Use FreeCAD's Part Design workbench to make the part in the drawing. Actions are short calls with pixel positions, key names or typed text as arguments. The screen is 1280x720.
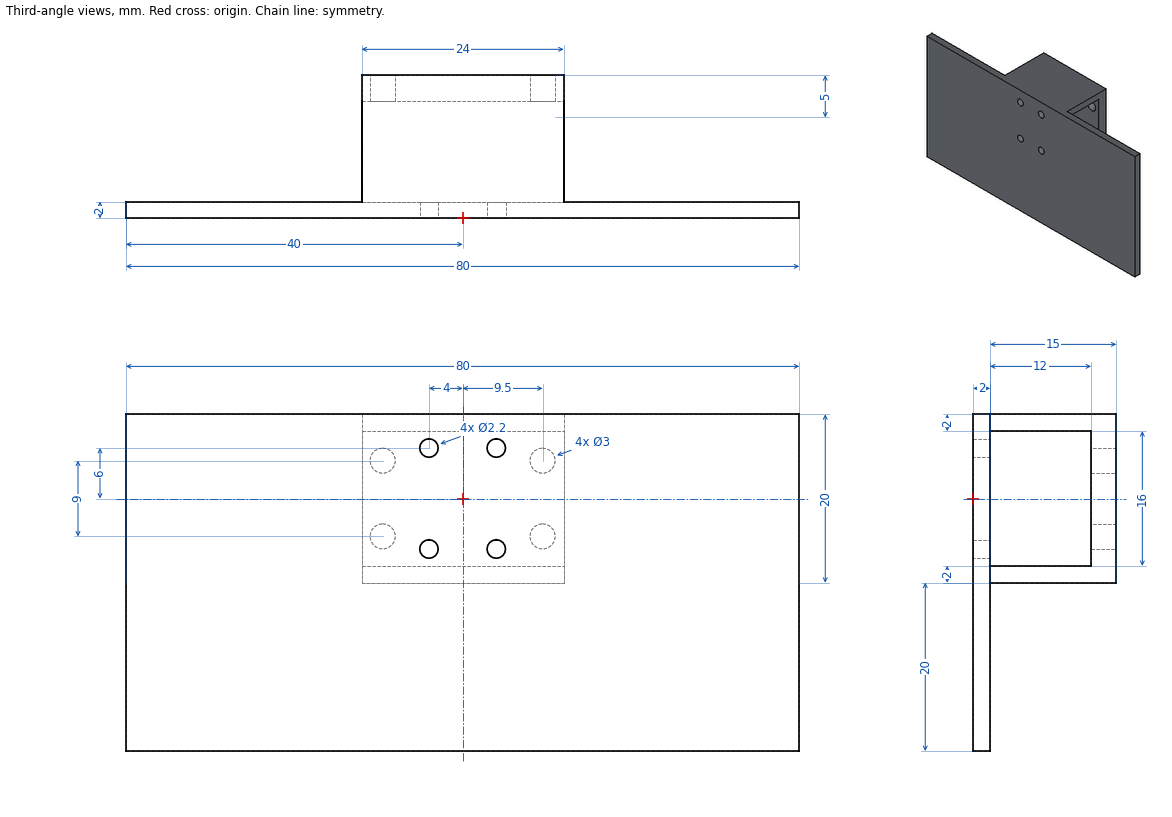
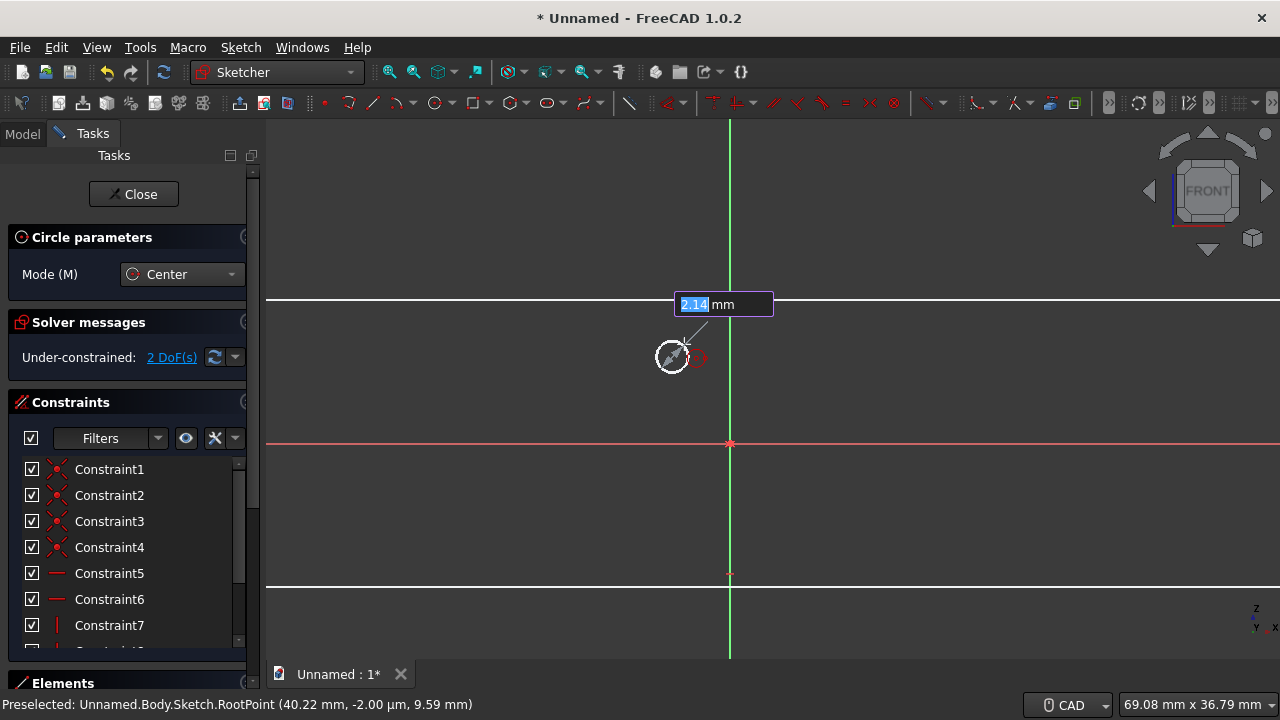
click(683, 344)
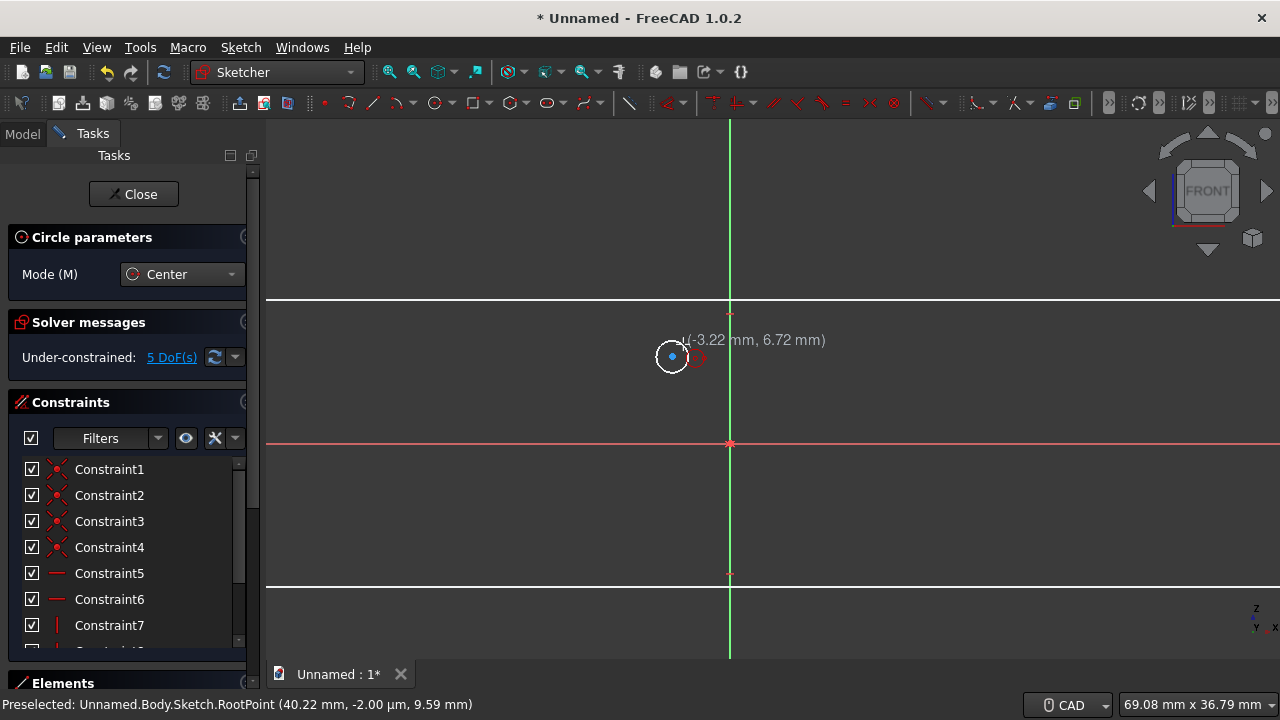
scroll(789, 356, up, 2)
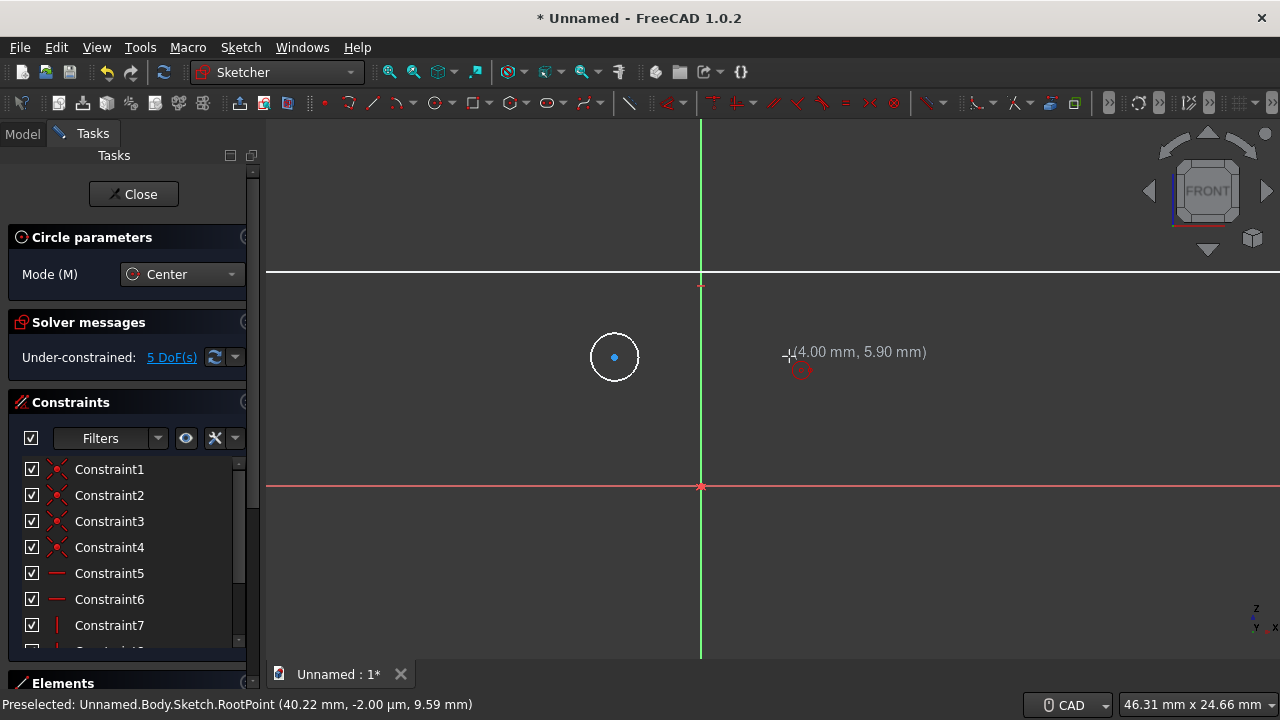
scroll(706, 347, down, 6)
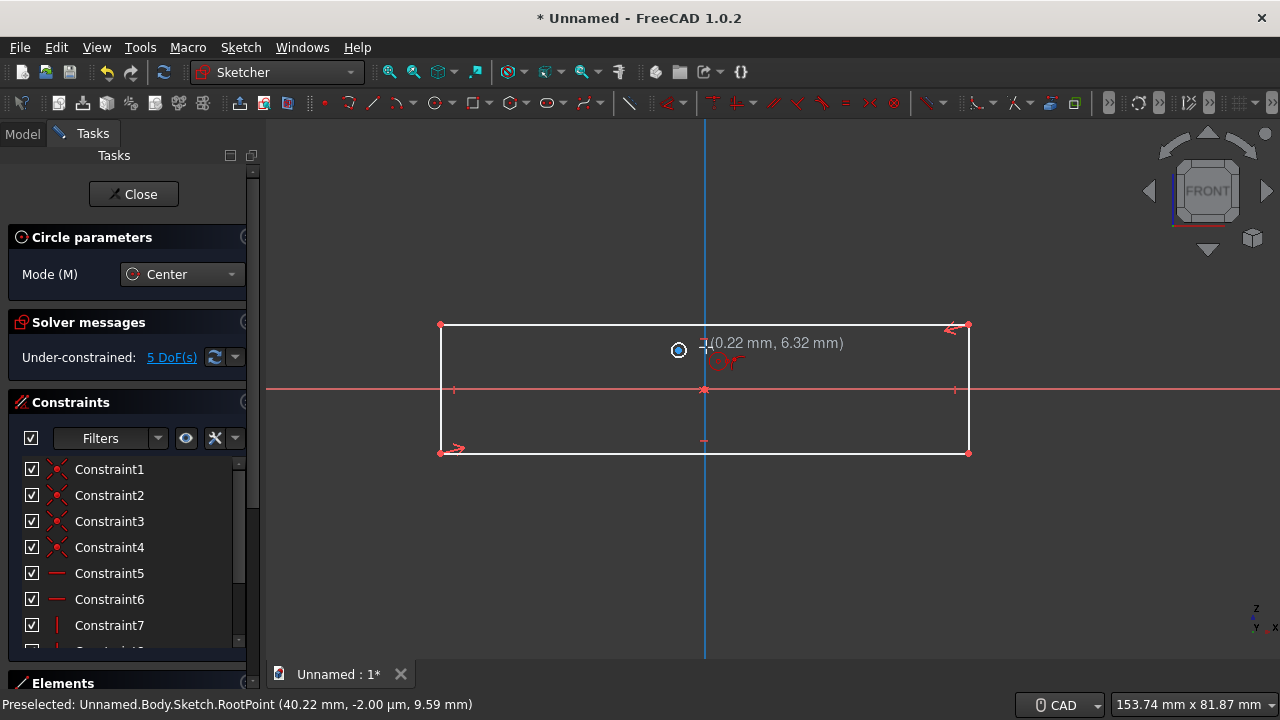
click(731, 350)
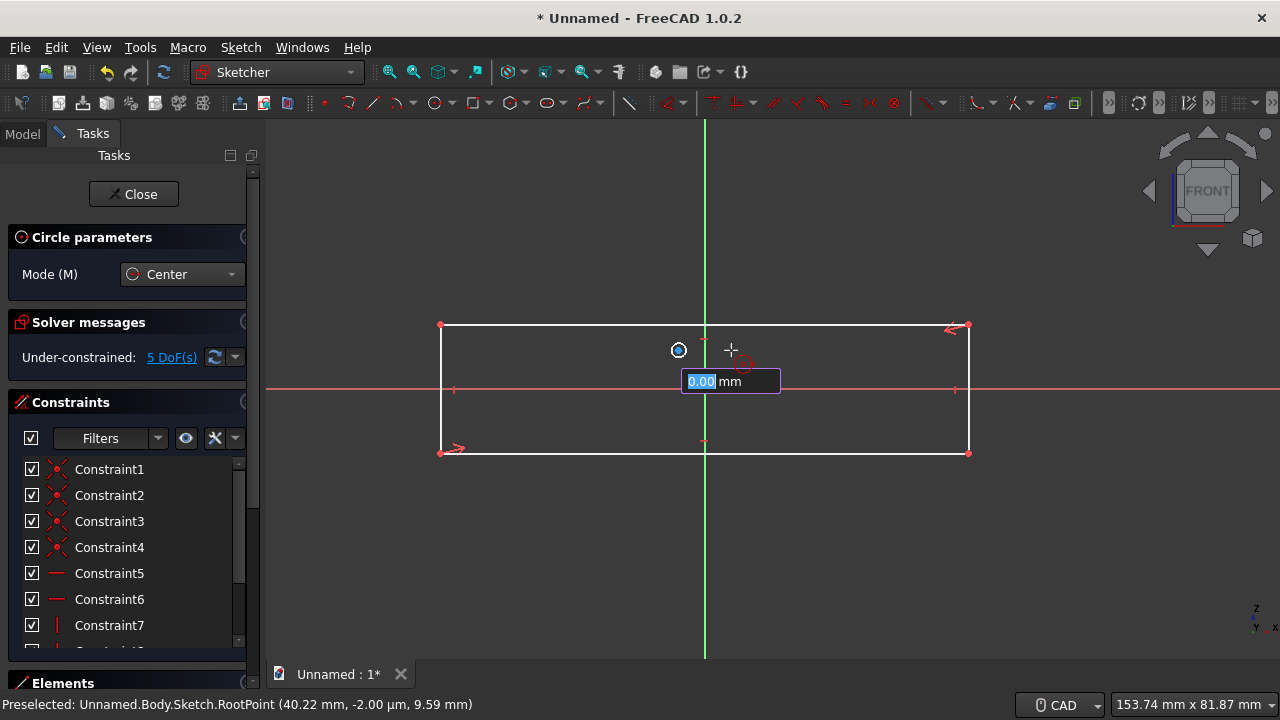
scroll(736, 345, up, 4)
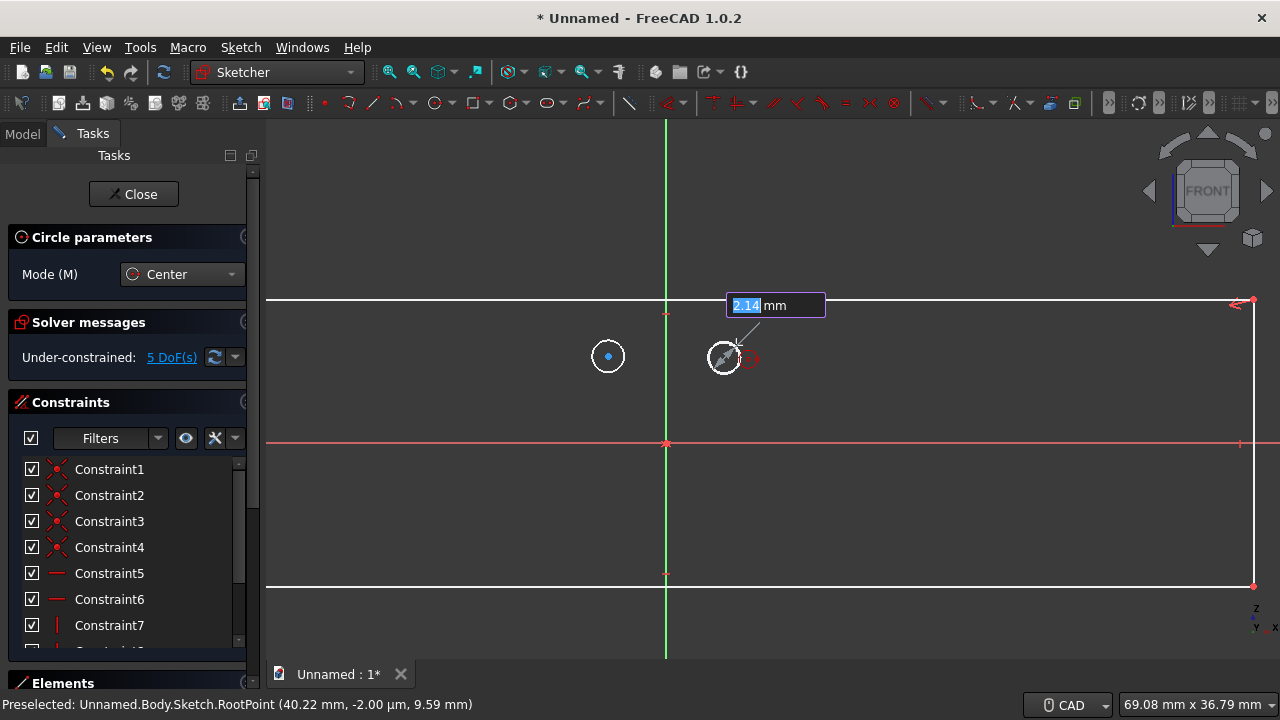
click(736, 344)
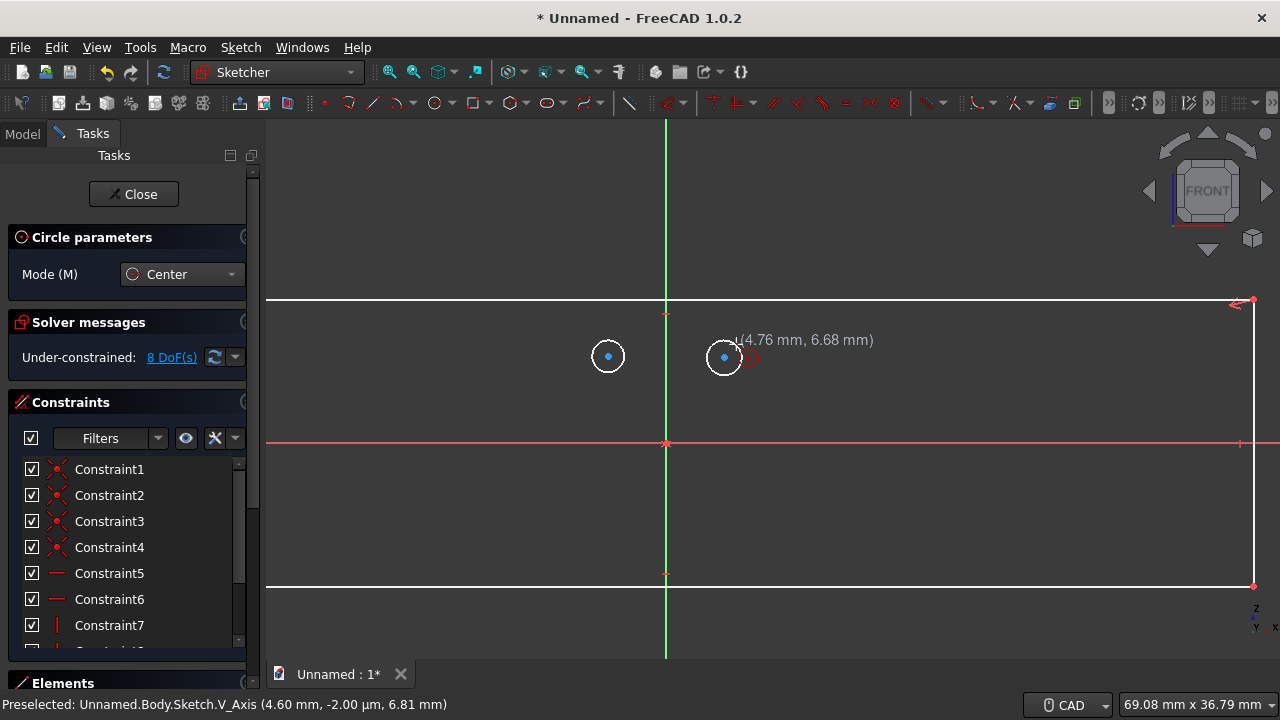
scroll(607, 531, up, 2)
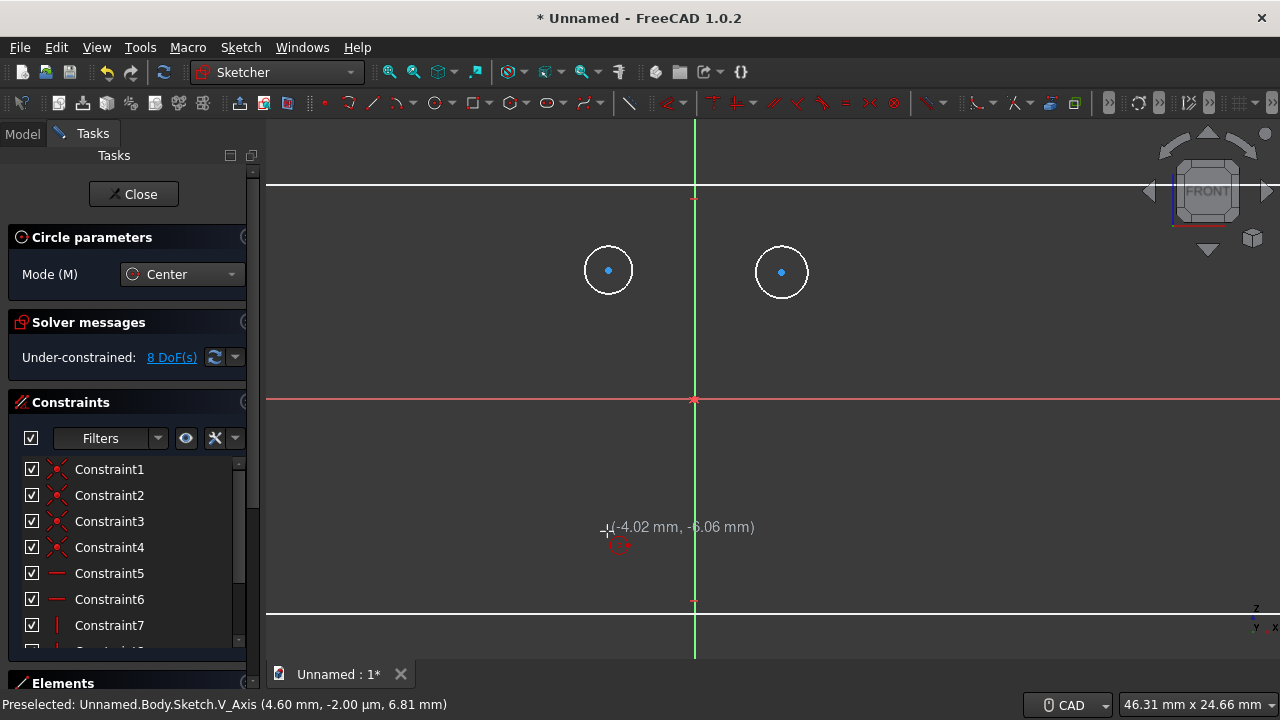
scroll(709, 384, down, 6)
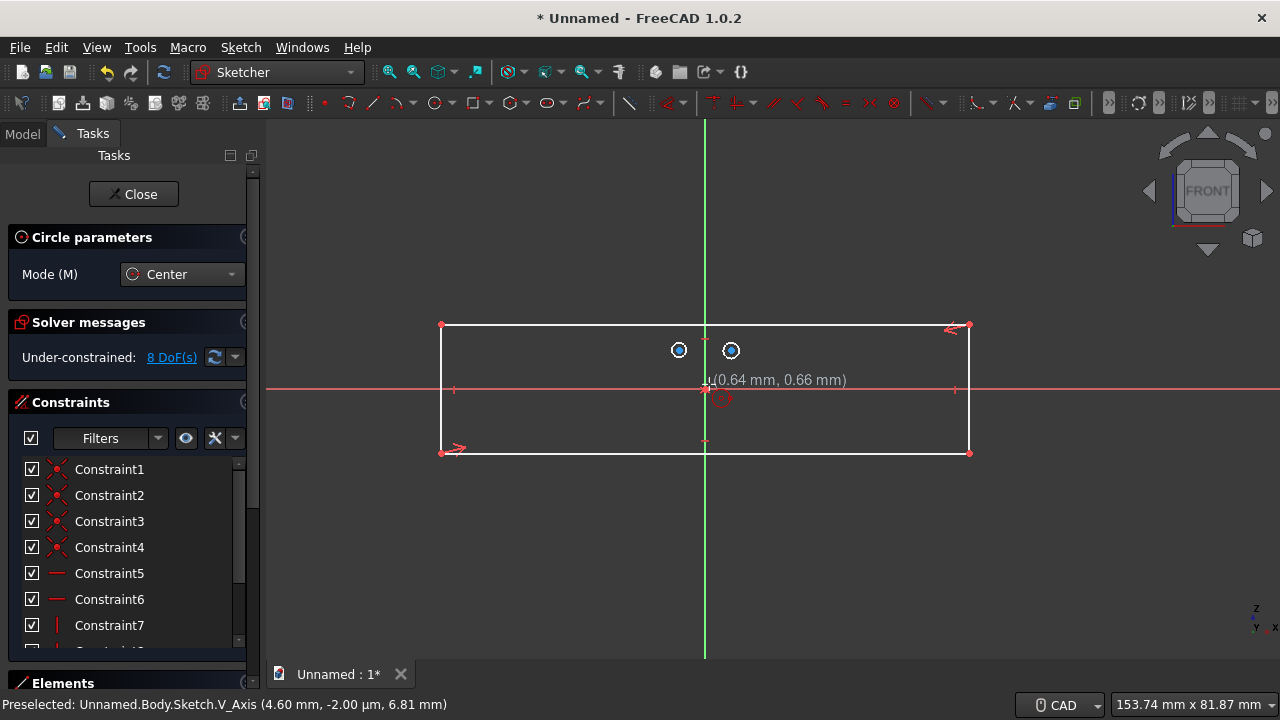
click(679, 429)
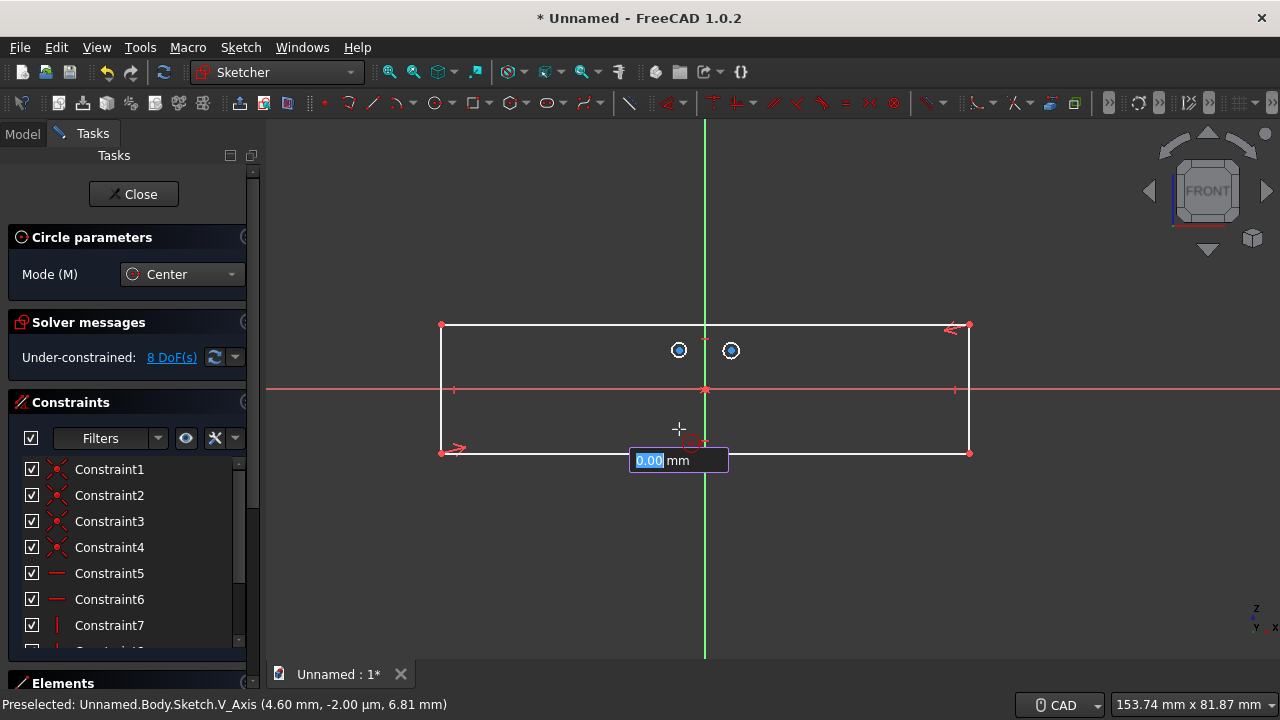
scroll(684, 423, up, 4)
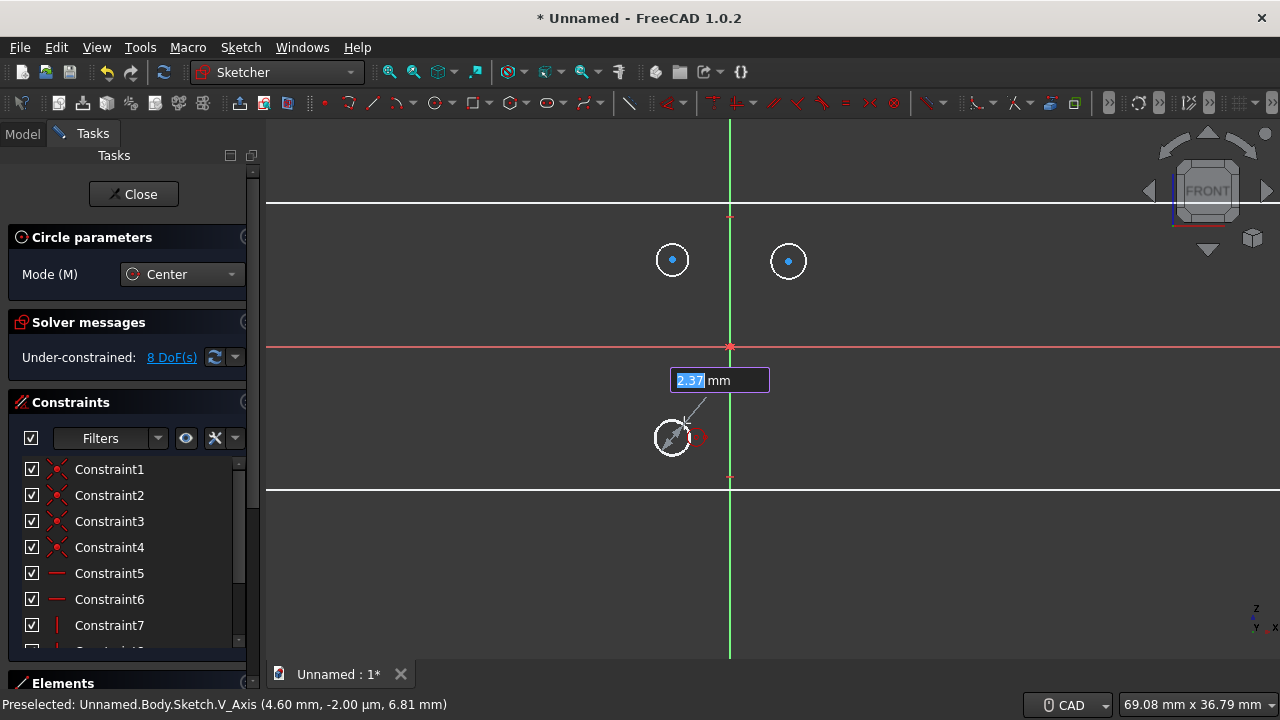
click(683, 423)